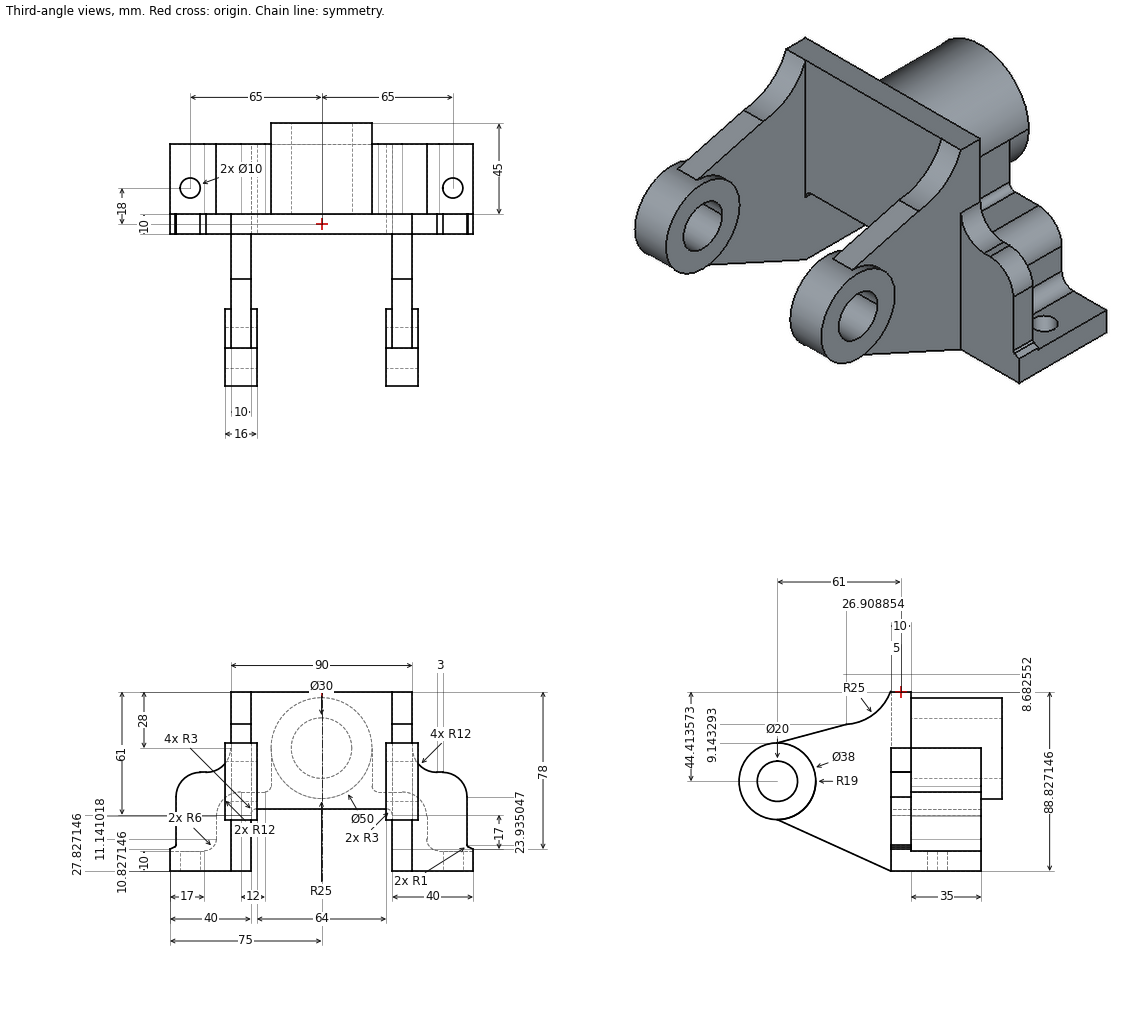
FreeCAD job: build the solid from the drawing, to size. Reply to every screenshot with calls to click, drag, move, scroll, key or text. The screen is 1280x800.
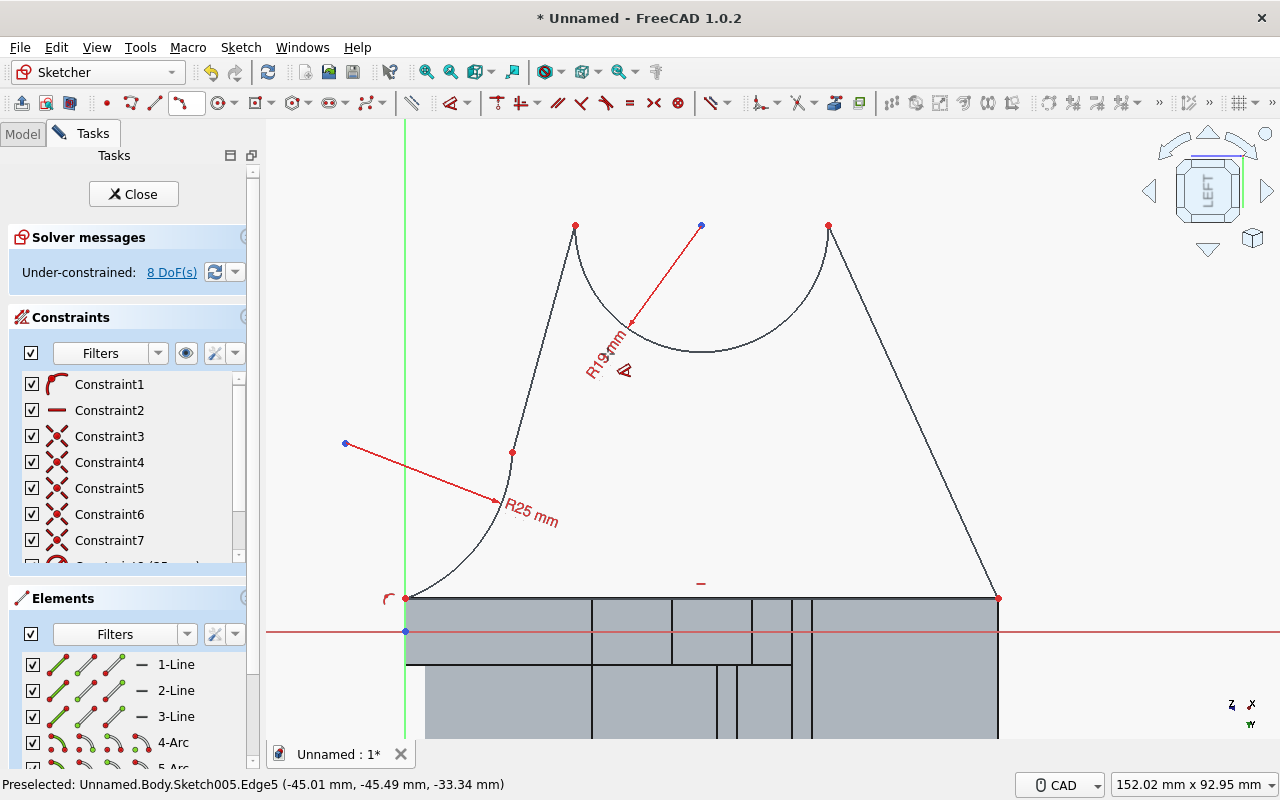
click(405, 599)
click(371, 615)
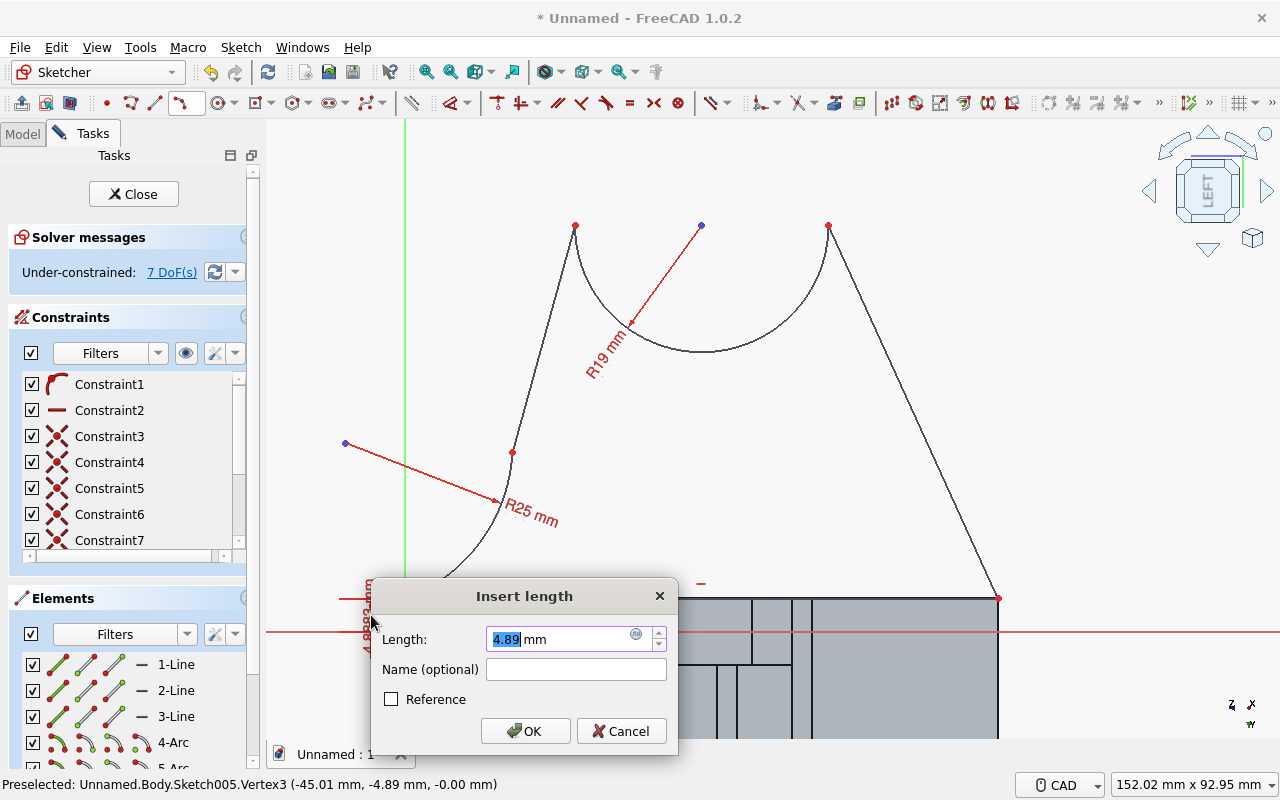
text(5)
key(Return)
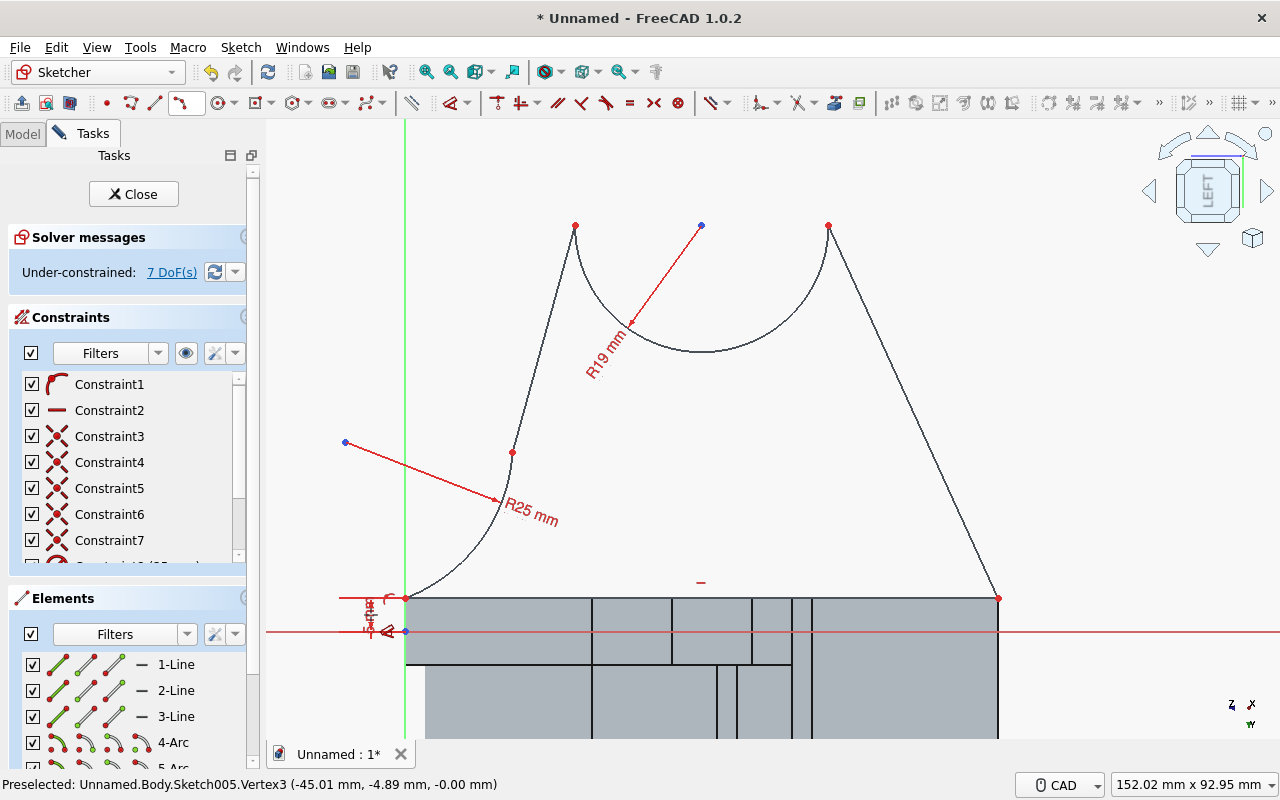
click(575, 226)
click(371, 429)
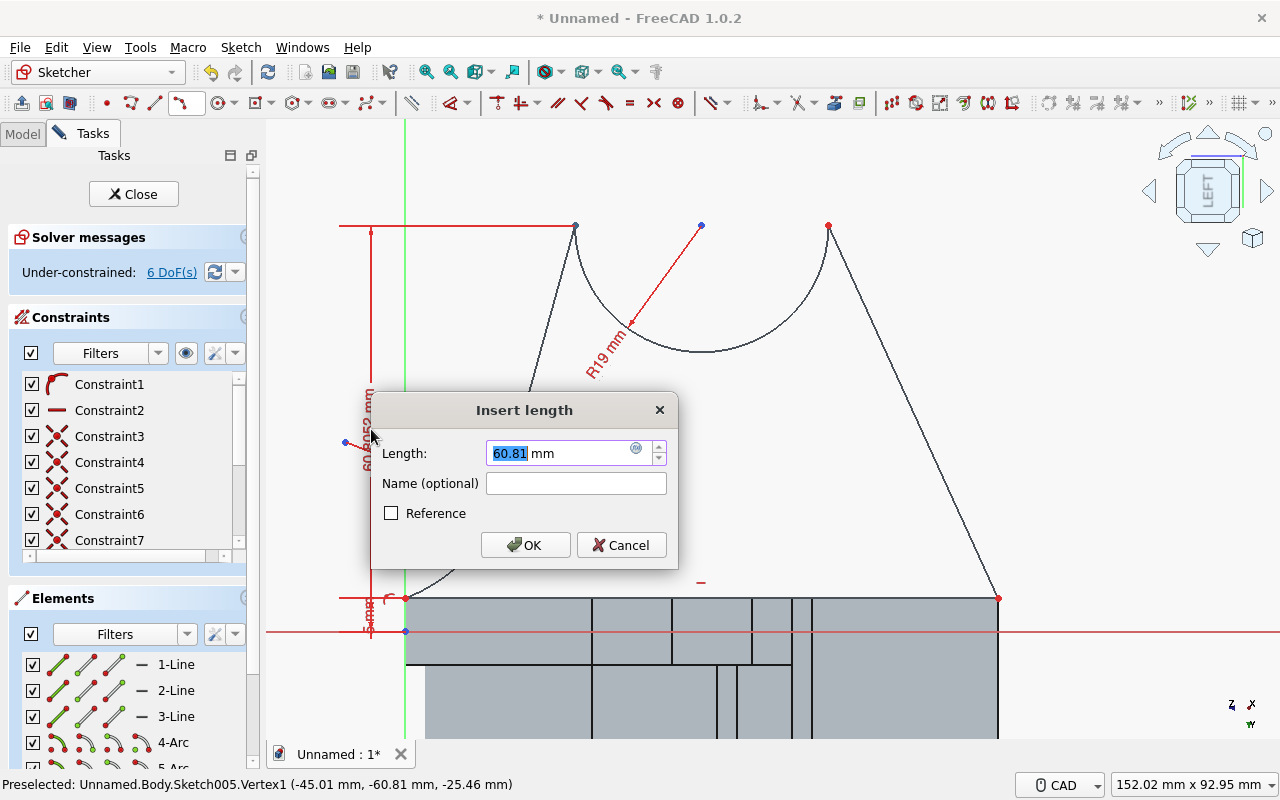
text(61)
key(Return)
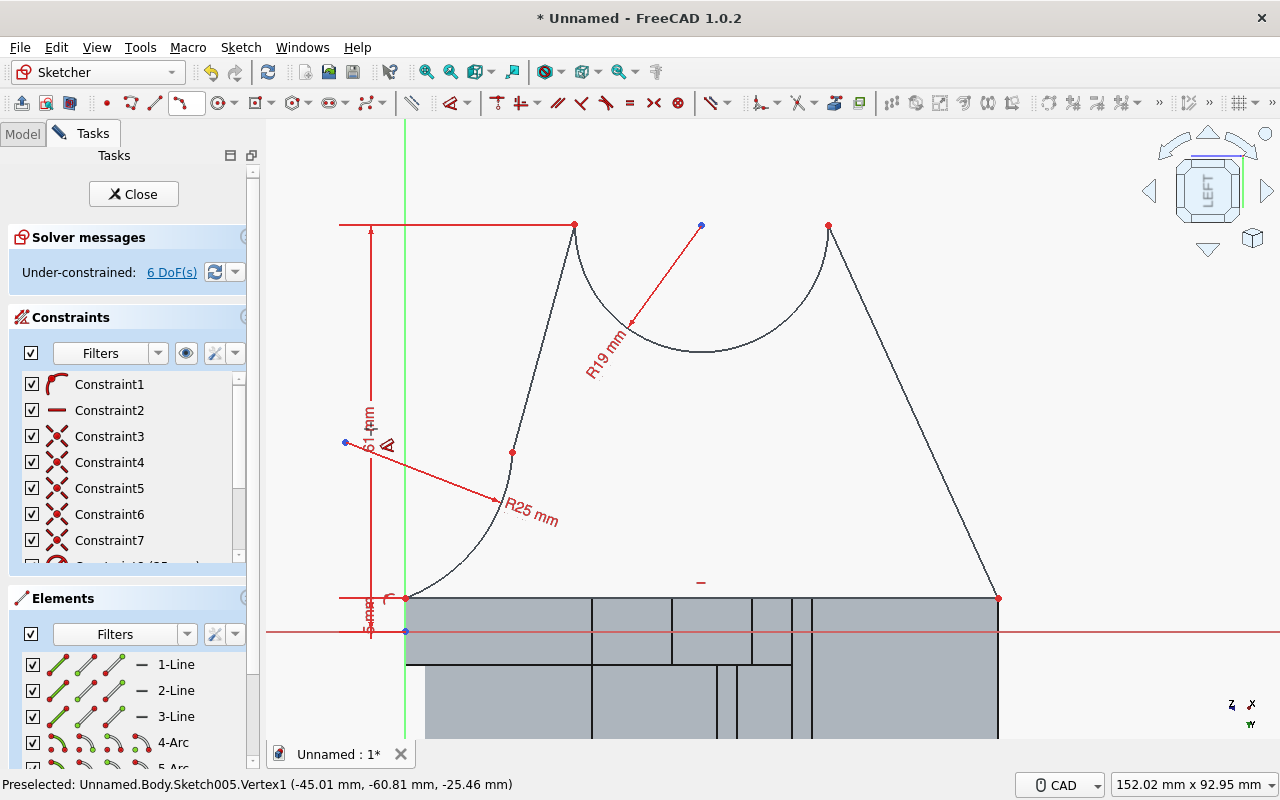
click(828, 226)
click(371, 336)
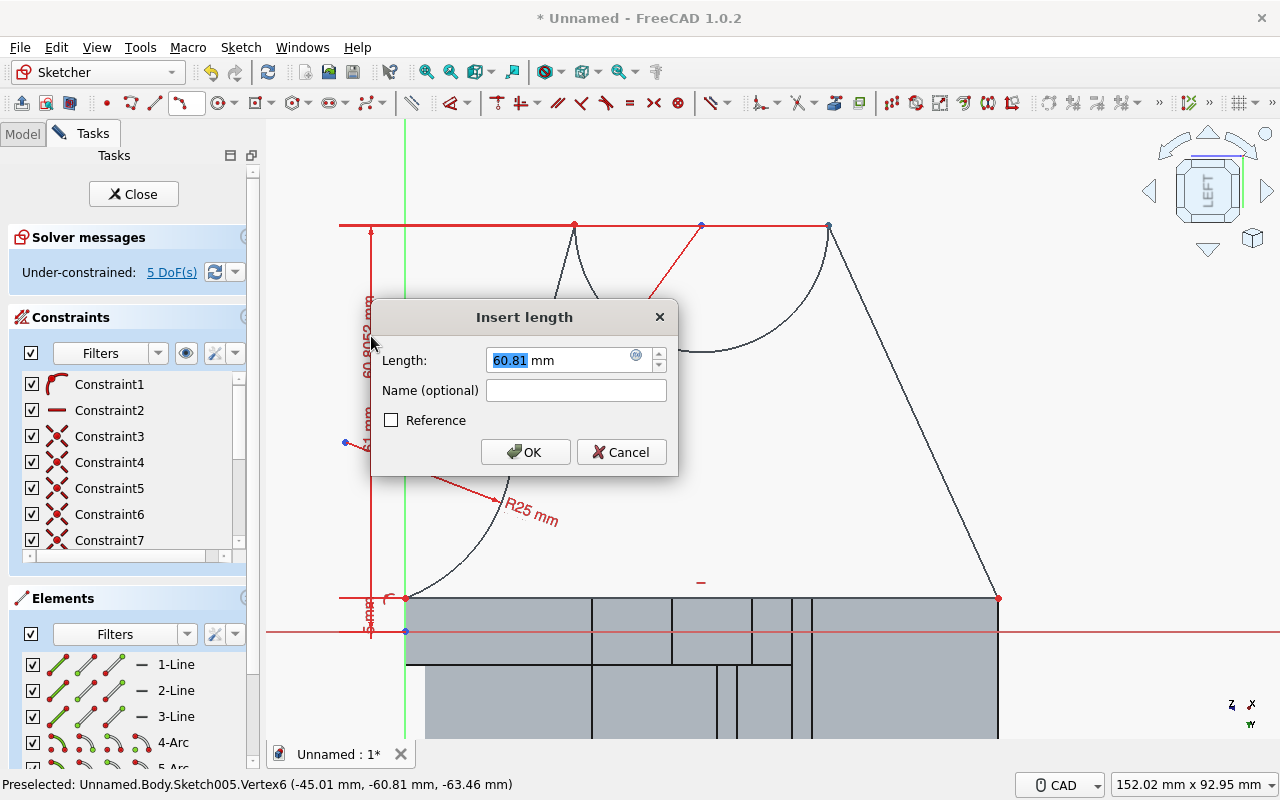
text(61)
key(Return)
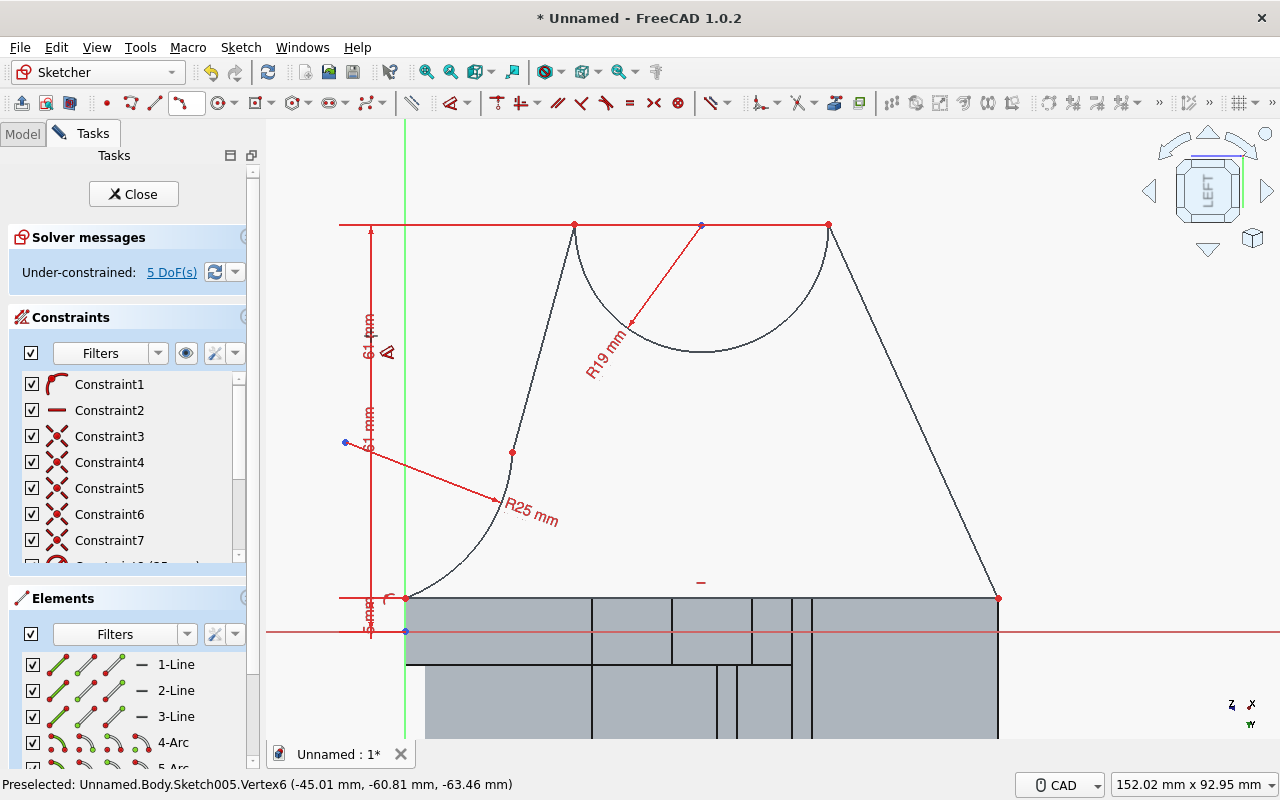
click(702, 226)
click(371, 522)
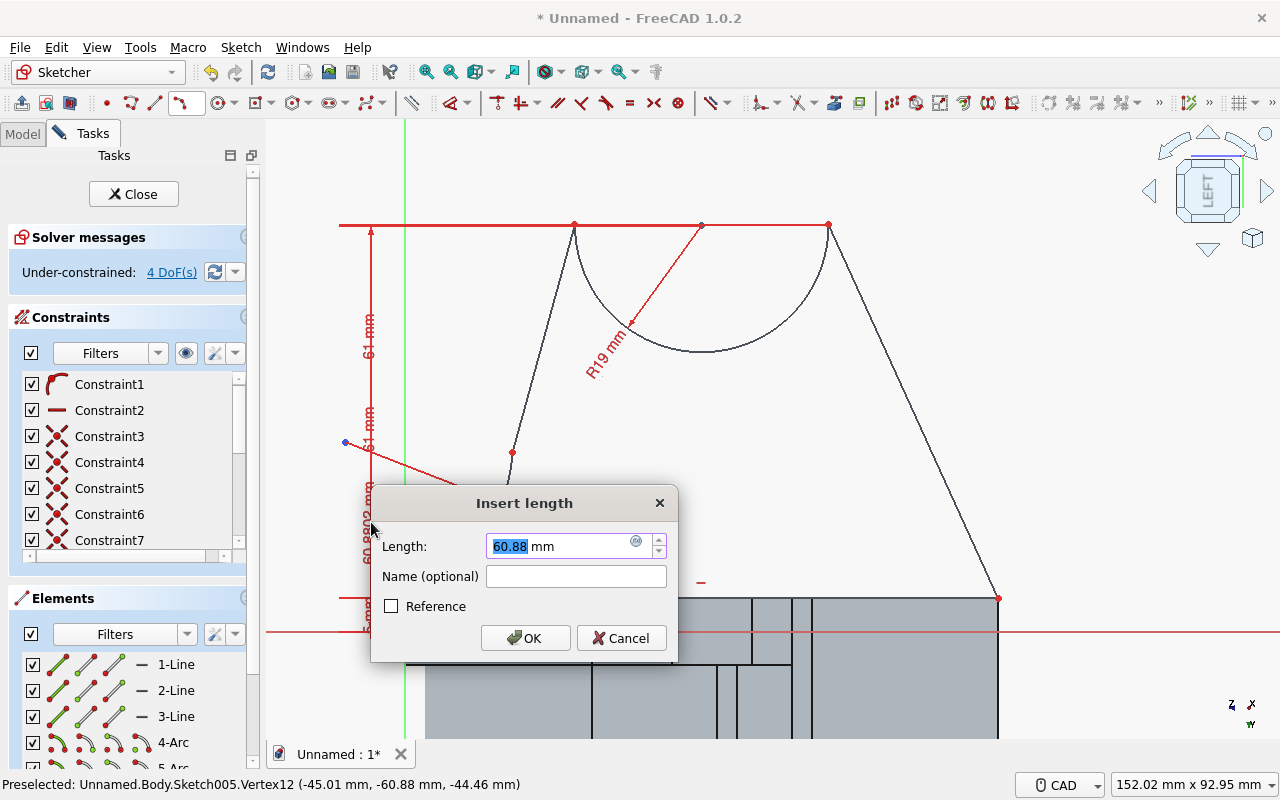
text(61)
key(Return)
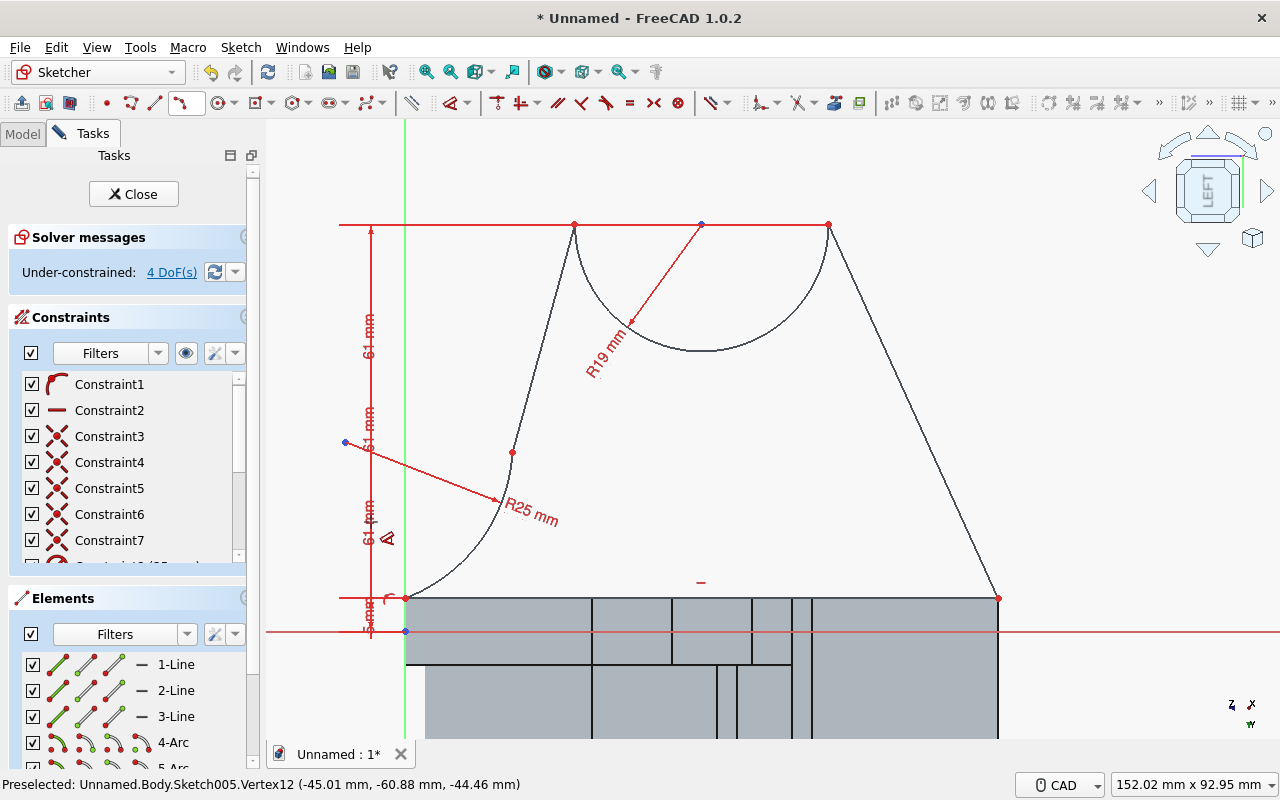
click(583, 598)
click(702, 564)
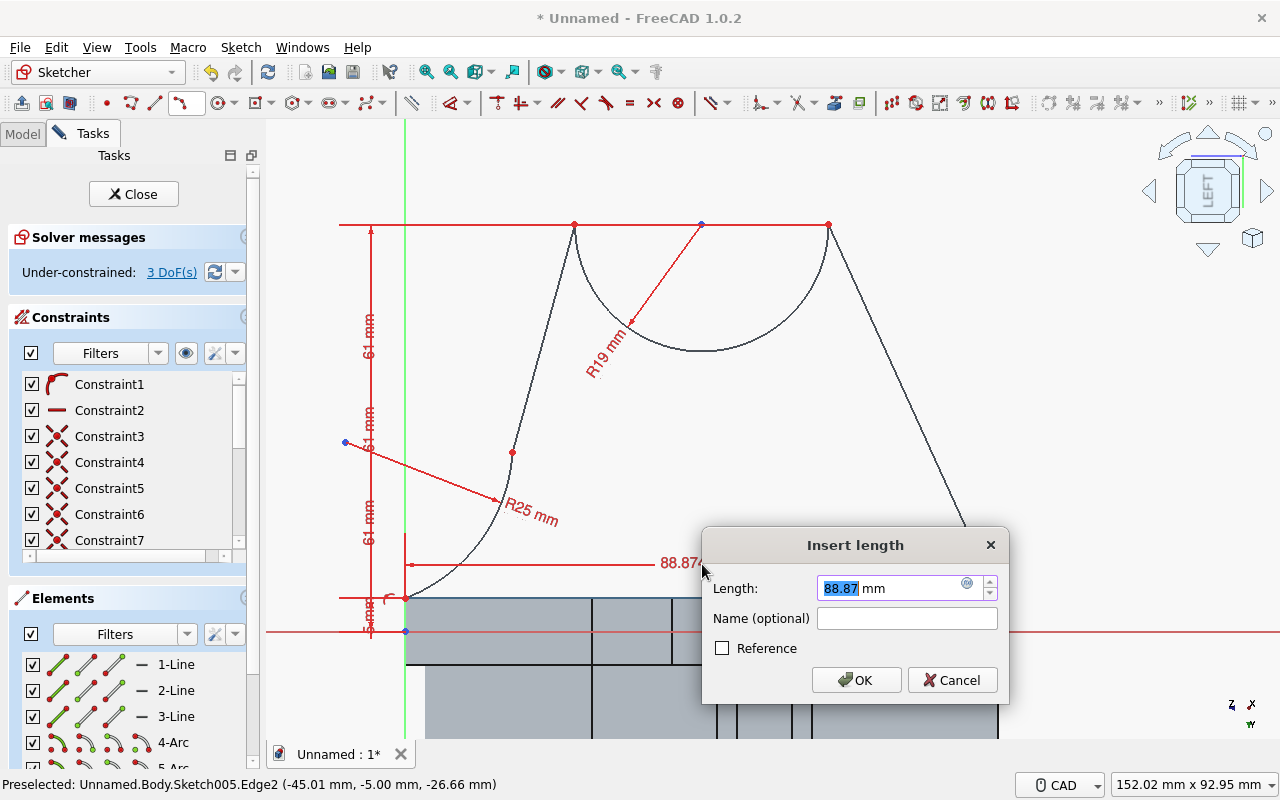
text(88.827146)
key(Return)